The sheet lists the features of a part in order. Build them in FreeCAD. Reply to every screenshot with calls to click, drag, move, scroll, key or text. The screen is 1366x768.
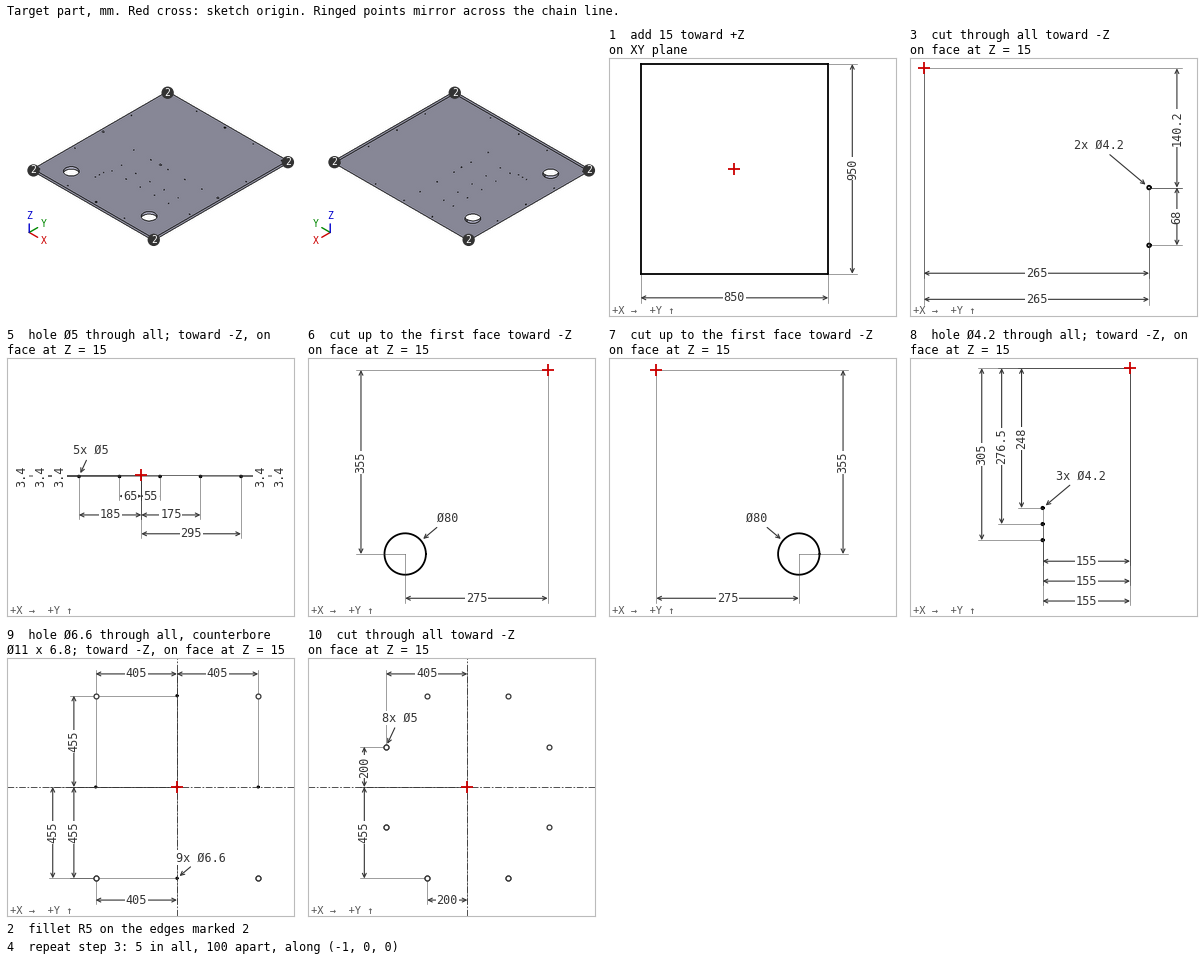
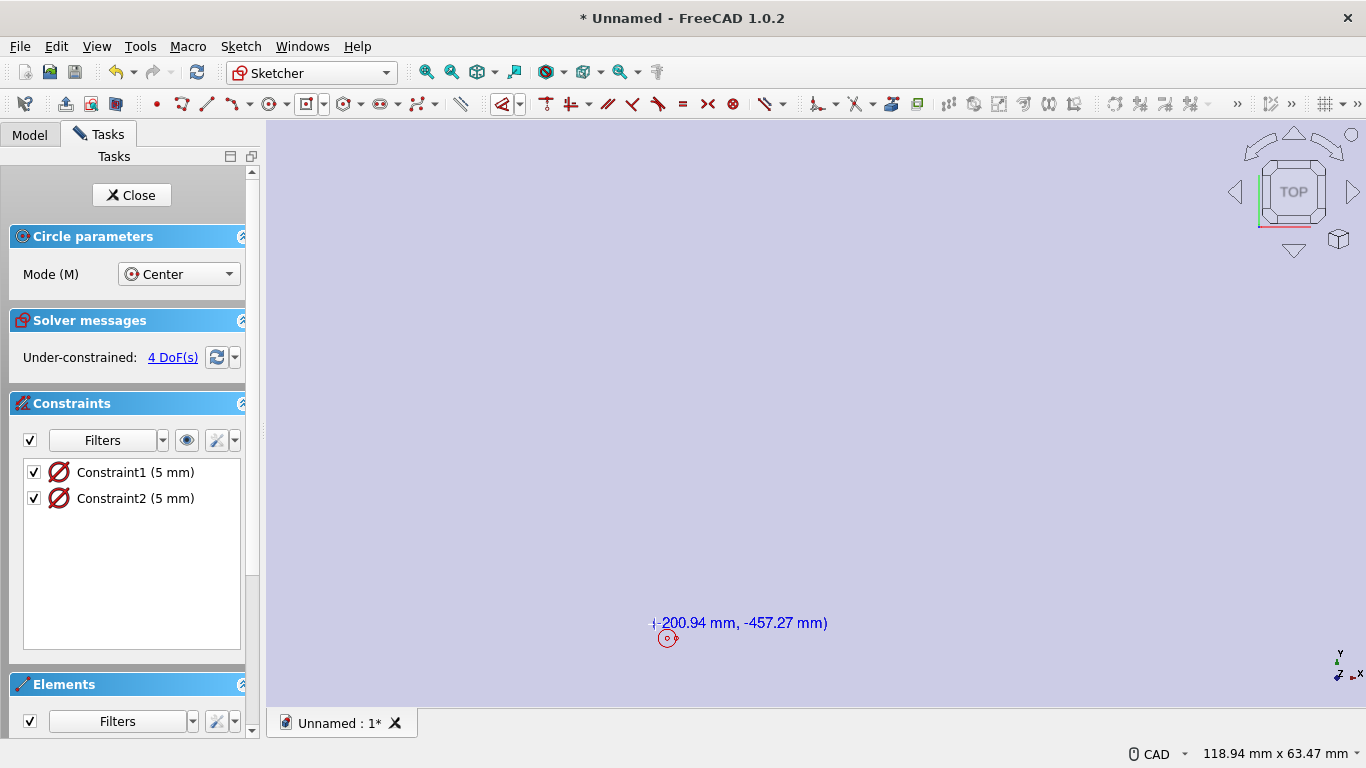
scroll(655, 624, down, 15)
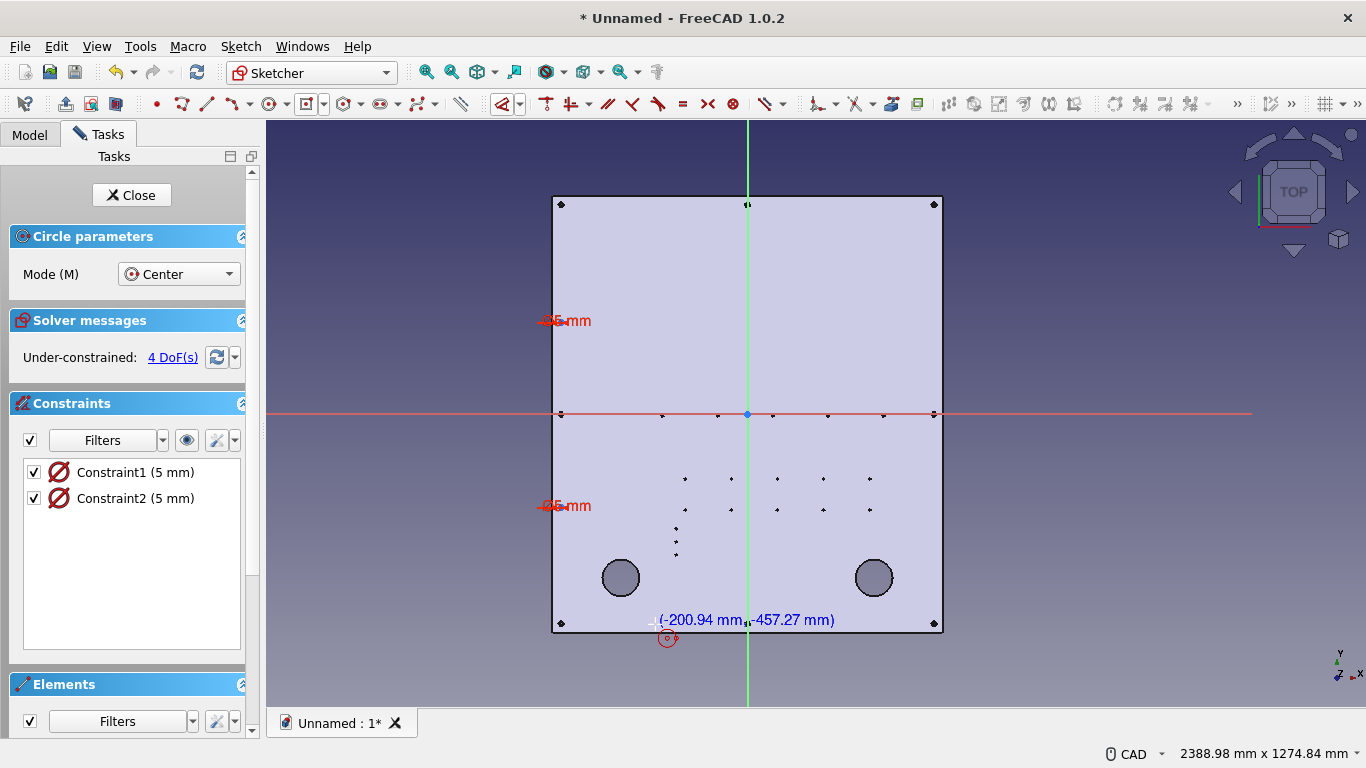
click(655, 624)
move(656, 623)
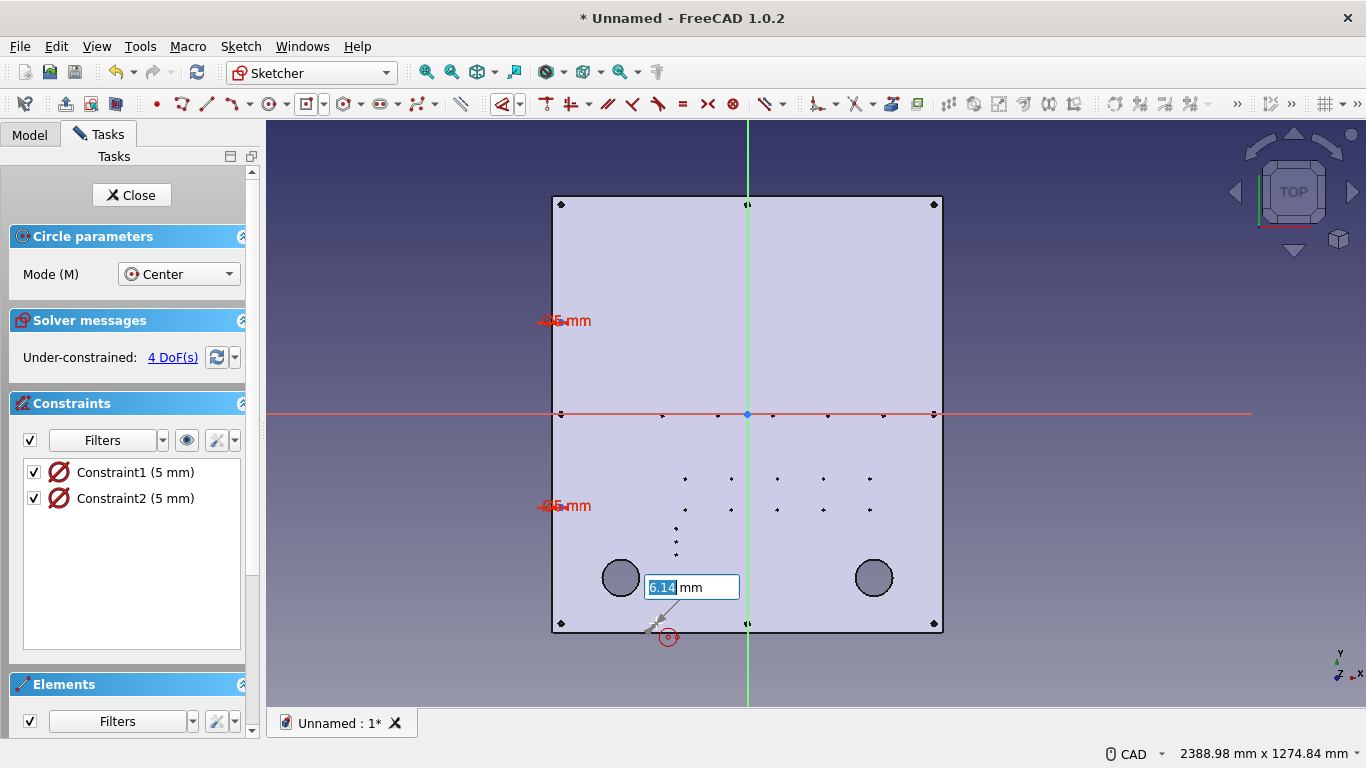
text(5)
key(Return)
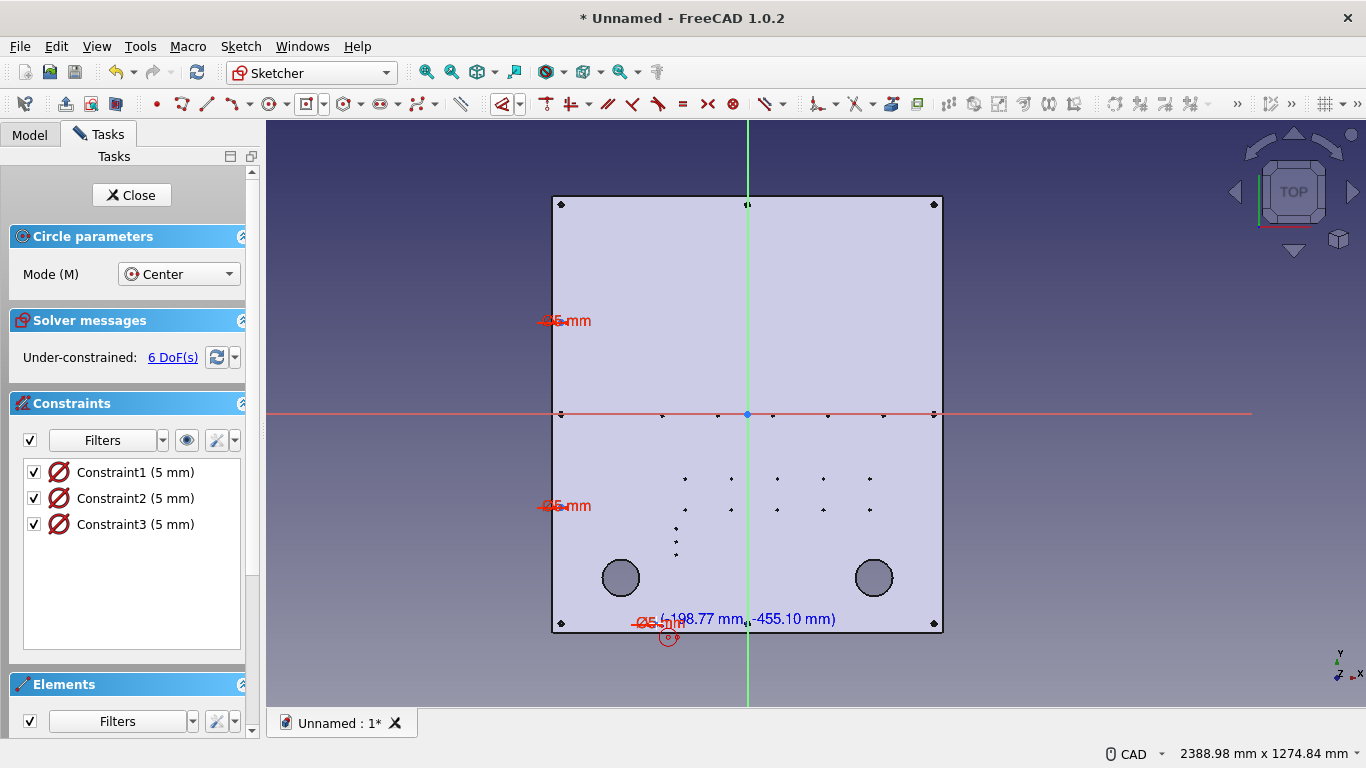
scroll(840, 624, up, 15)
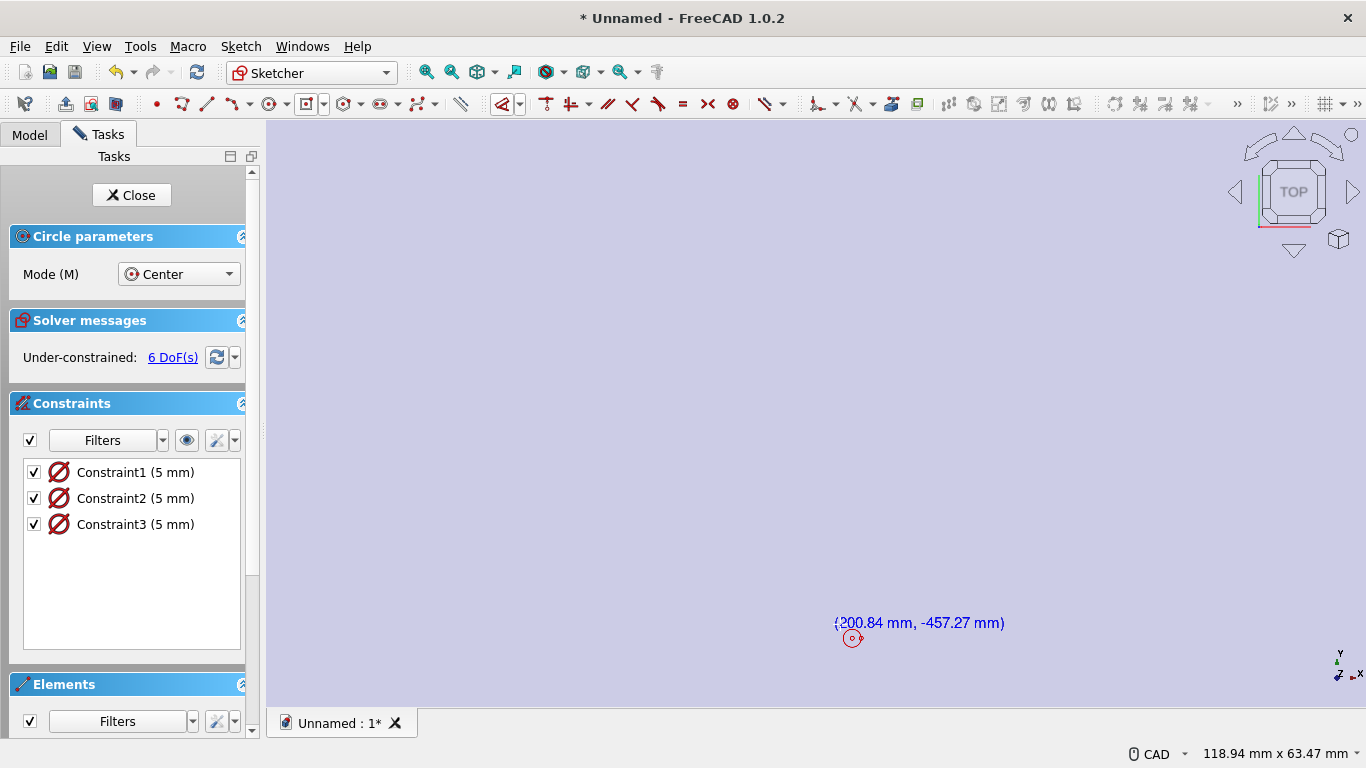
scroll(840, 624, down, 15)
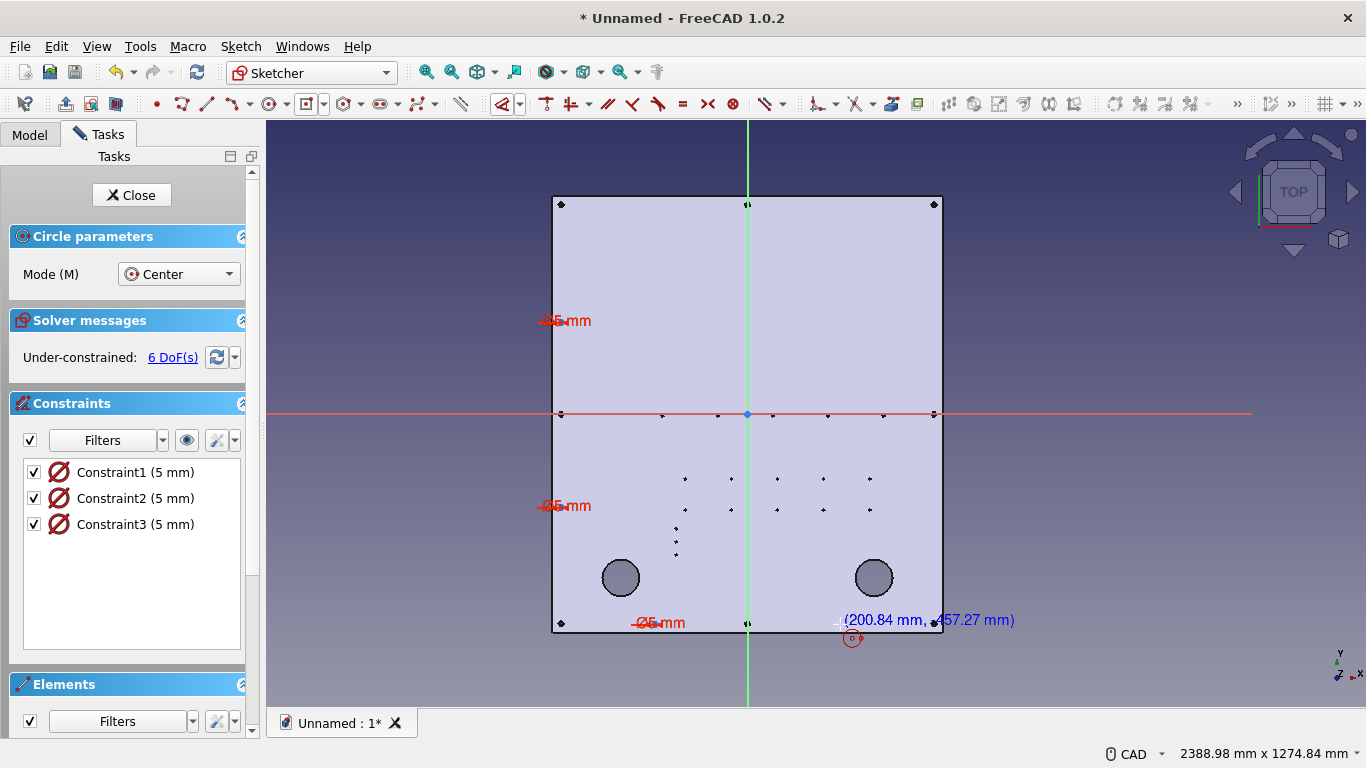
click(840, 624)
move(840, 623)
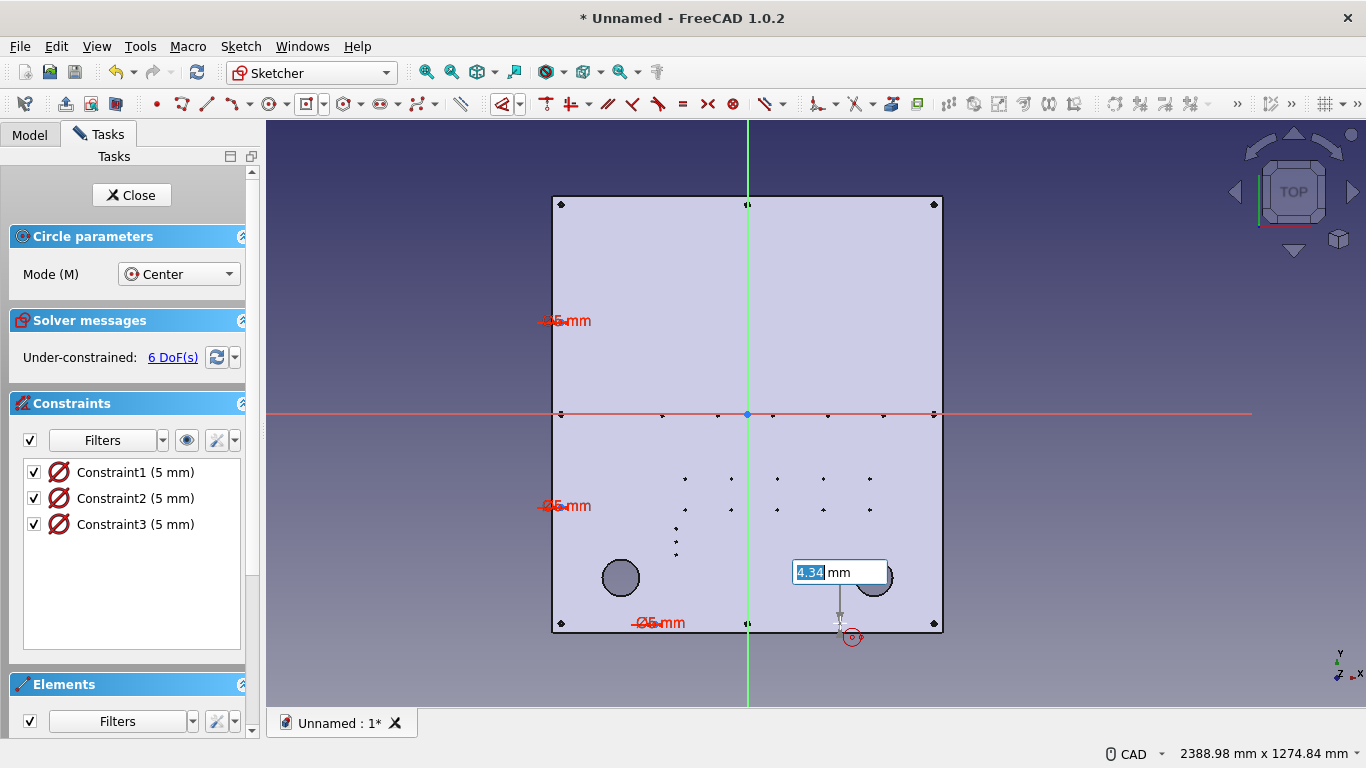
text(5)
key(Return)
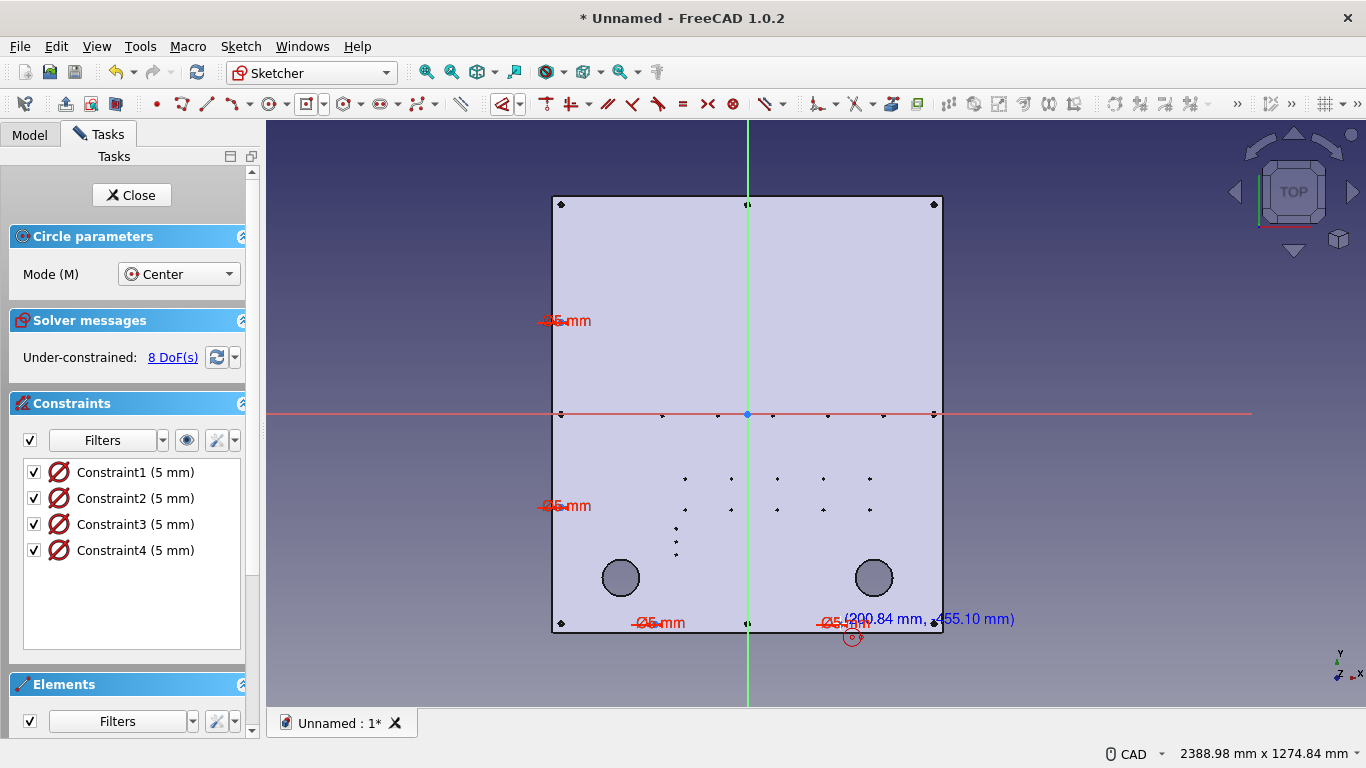
scroll(934, 507, up, 15)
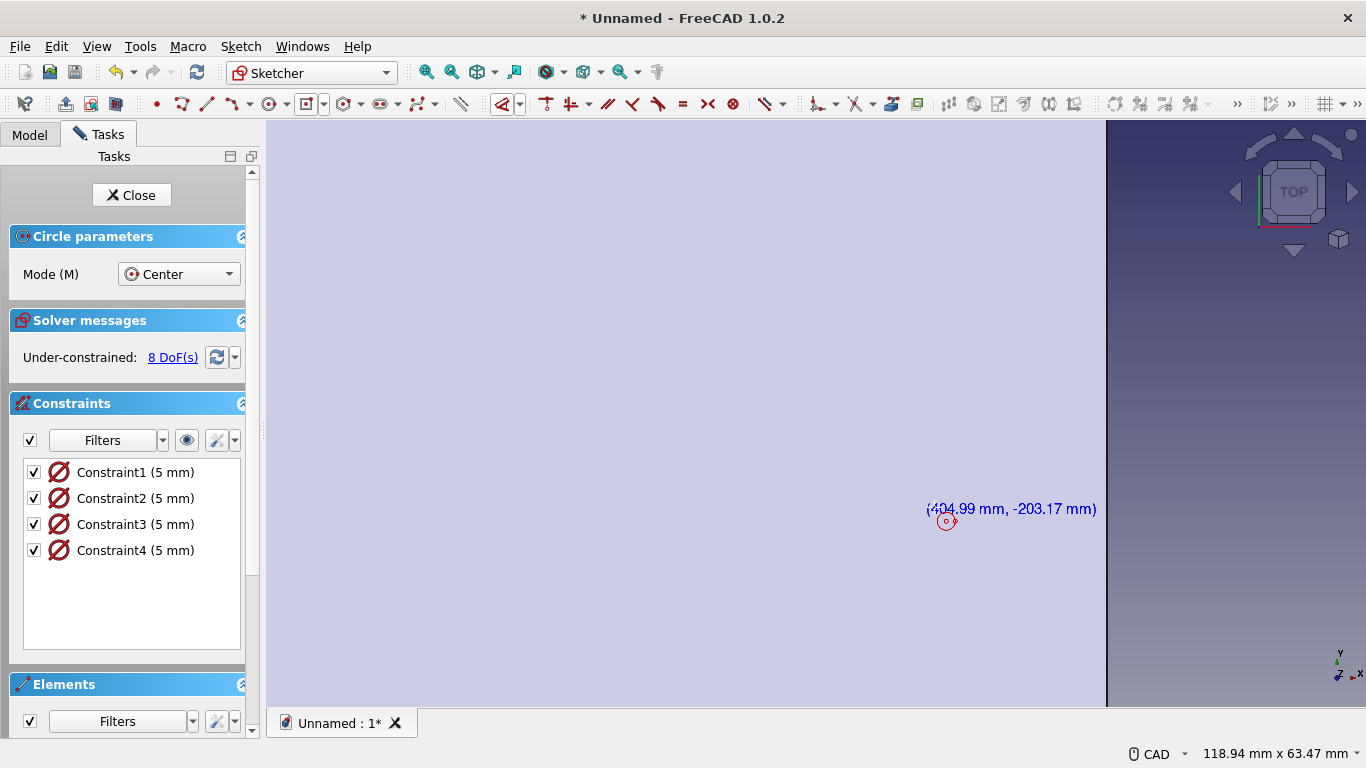
scroll(935, 507, down, 15)